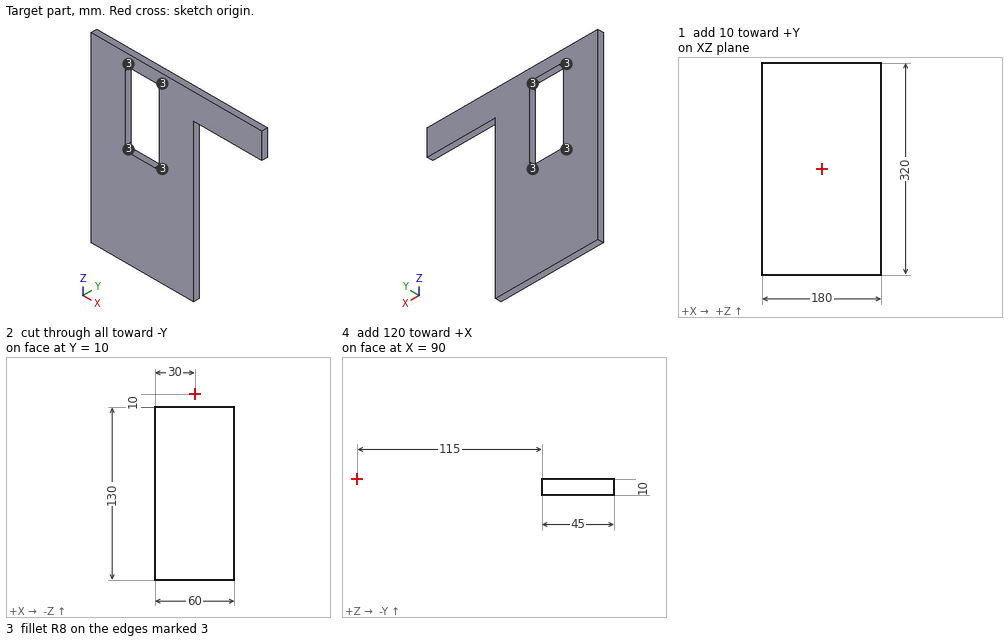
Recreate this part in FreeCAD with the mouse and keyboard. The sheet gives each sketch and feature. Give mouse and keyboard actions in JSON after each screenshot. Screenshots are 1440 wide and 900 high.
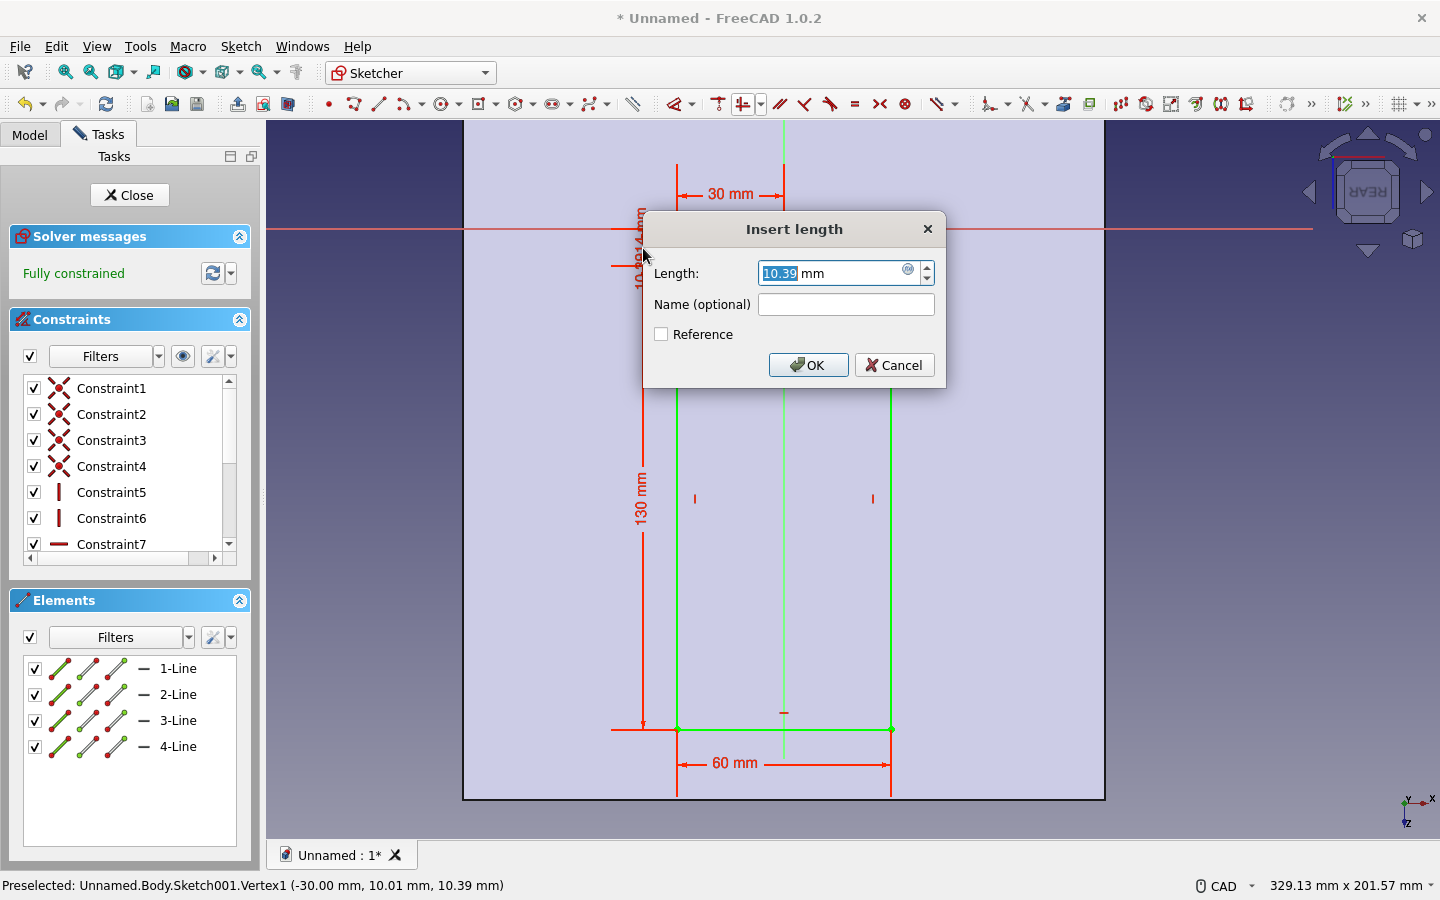
{"action": "type", "text": "10"}
{"action": "key", "text": "Return"}
{"action": "key", "text": "Escape"}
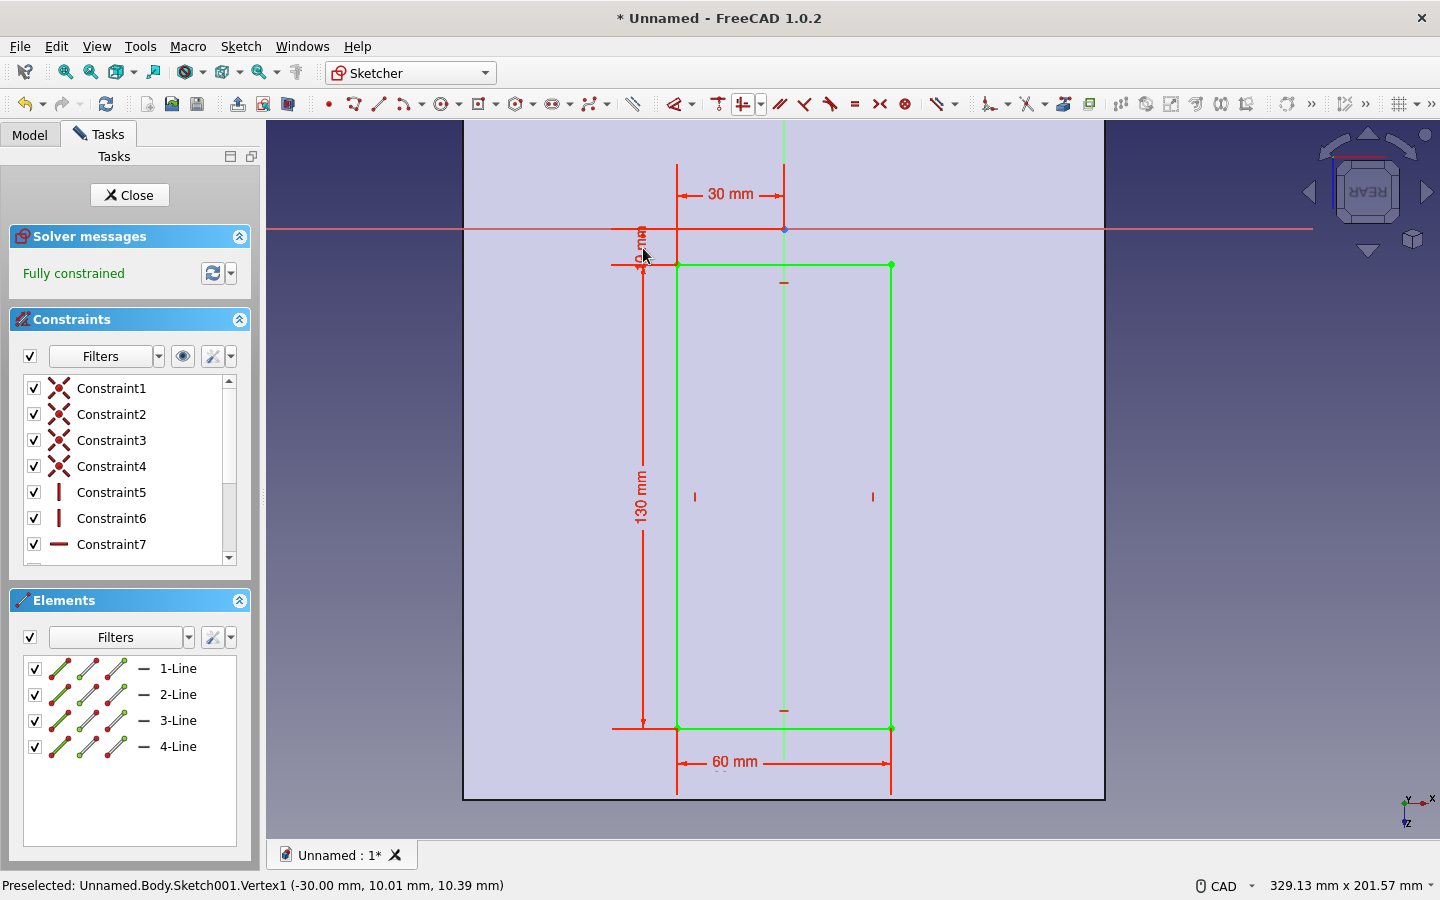
{"action": "left_click", "coordinate": [130, 195]}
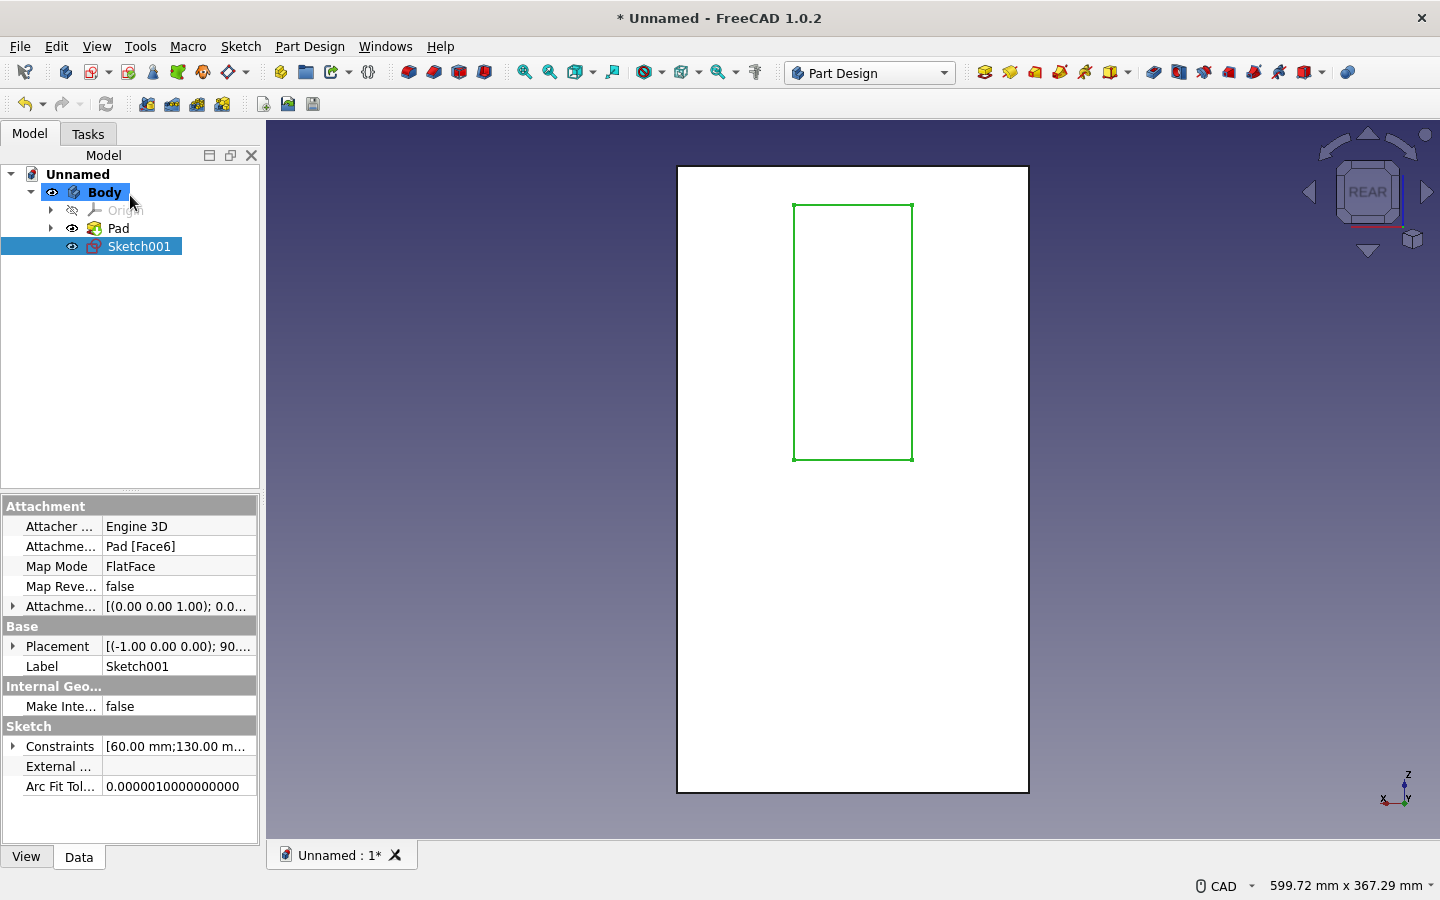
{"action": "left_click", "coordinate": [1154, 72]}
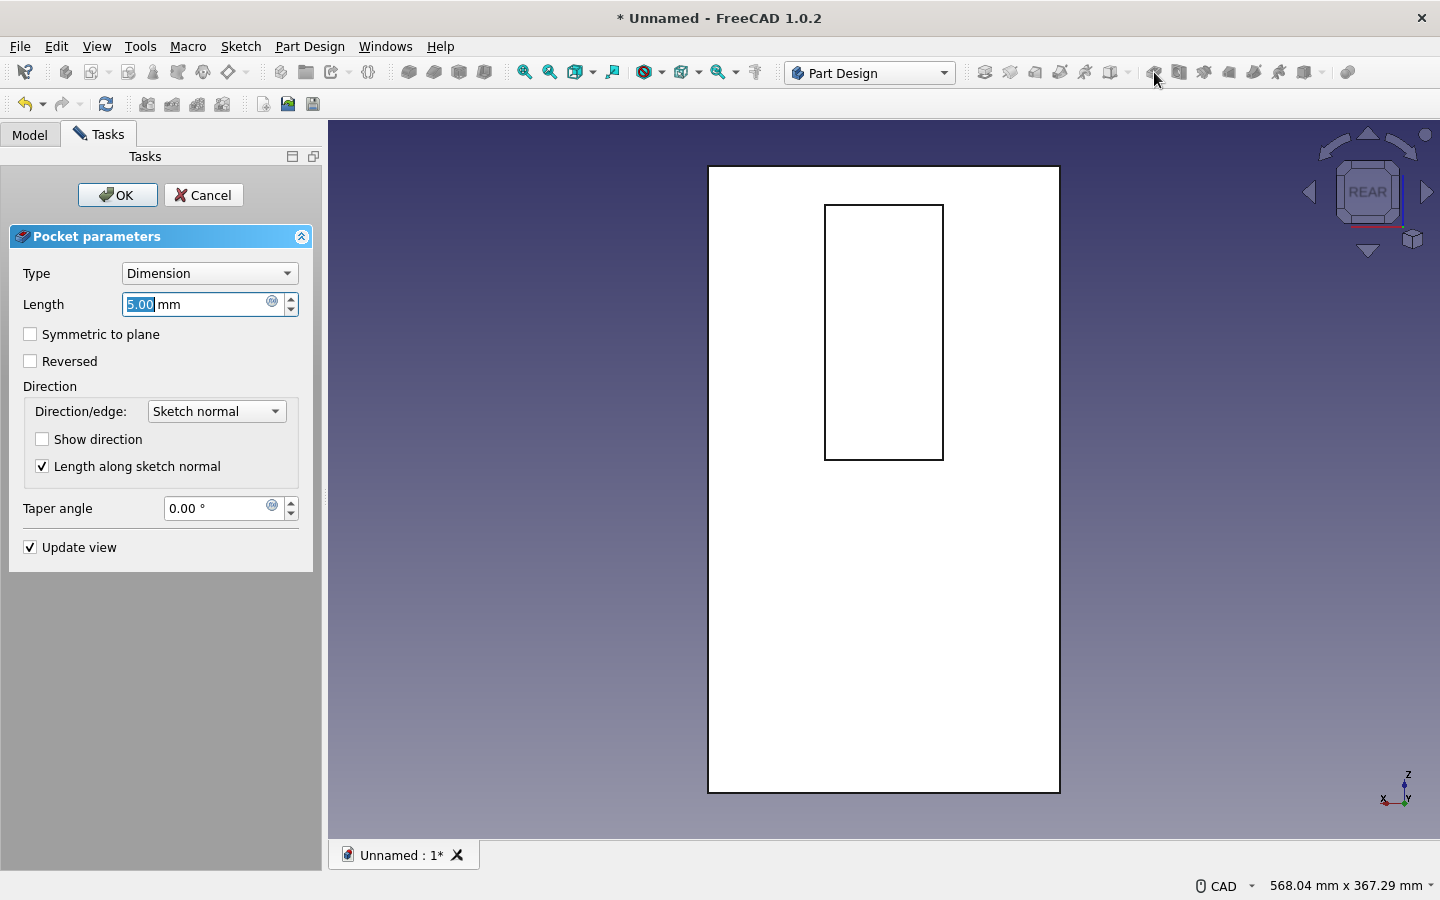
{"action": "left_click", "coordinate": [210, 274]}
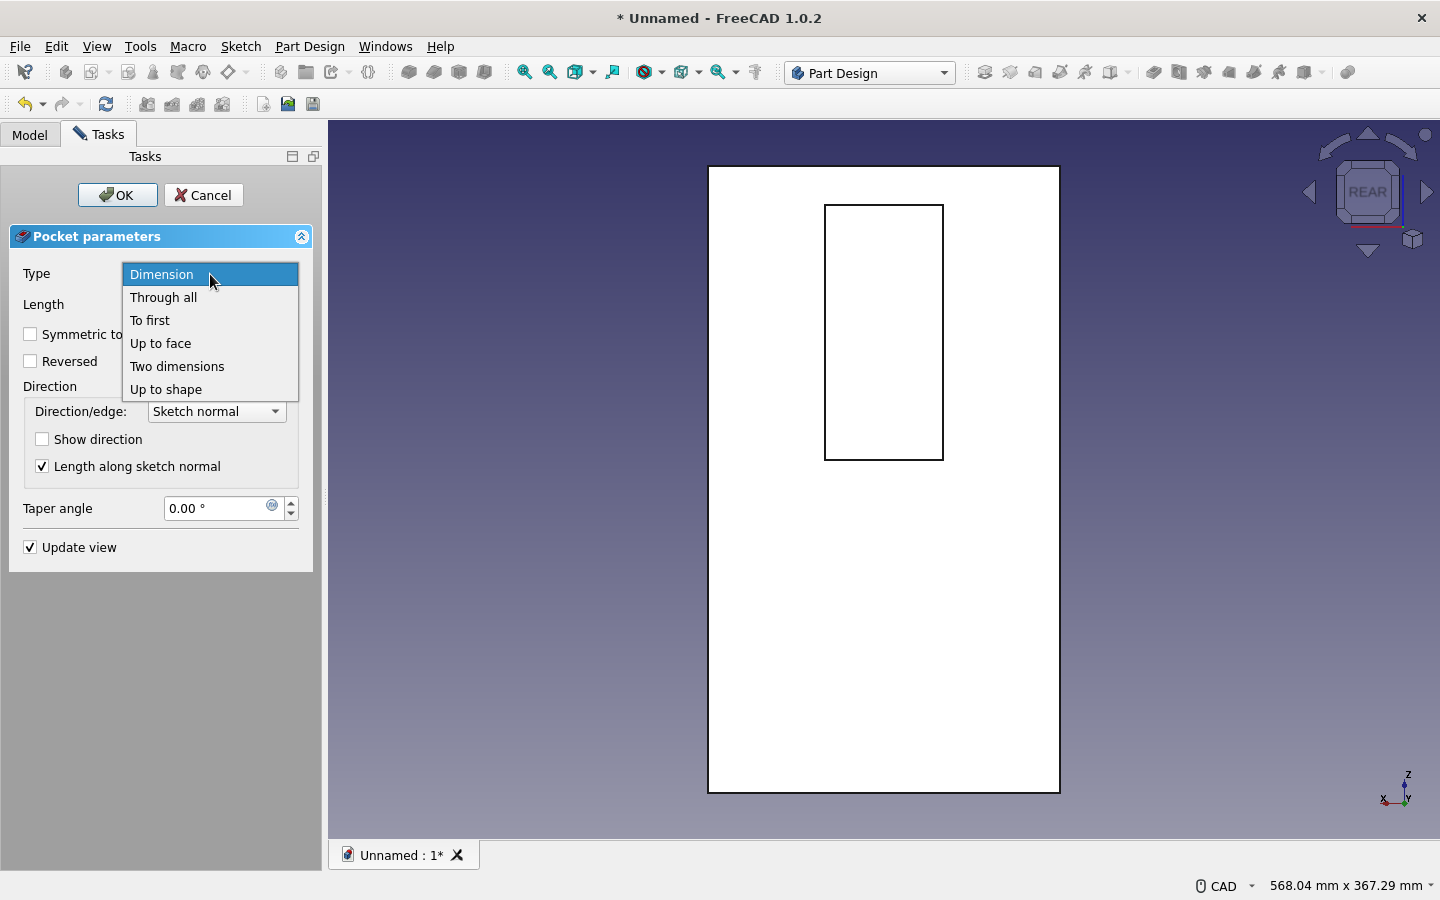
{"action": "left_click", "coordinate": [208, 298]}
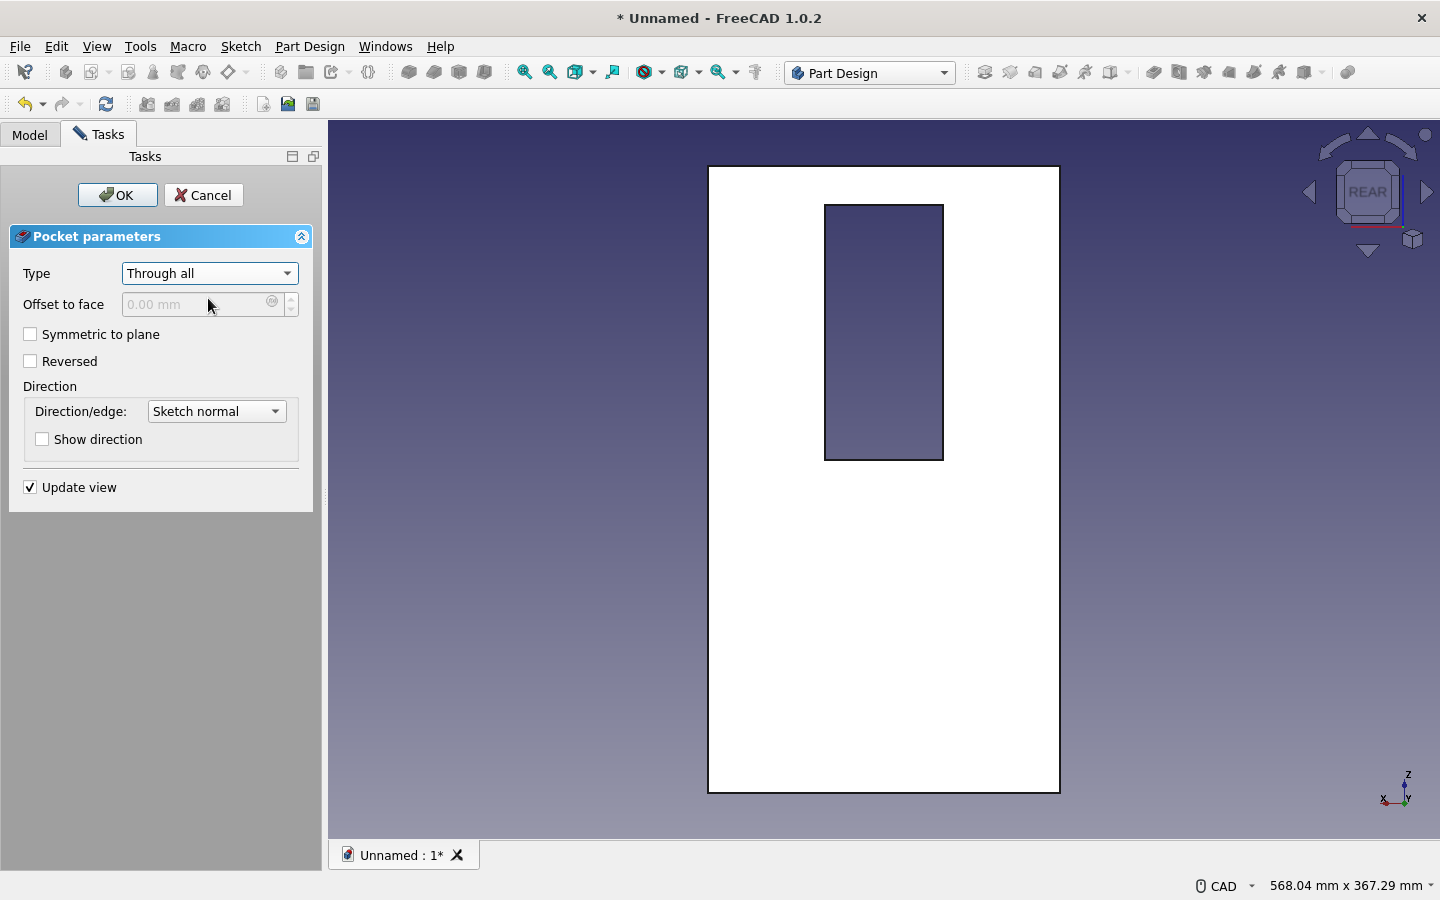
{"action": "left_click", "coordinate": [118, 195]}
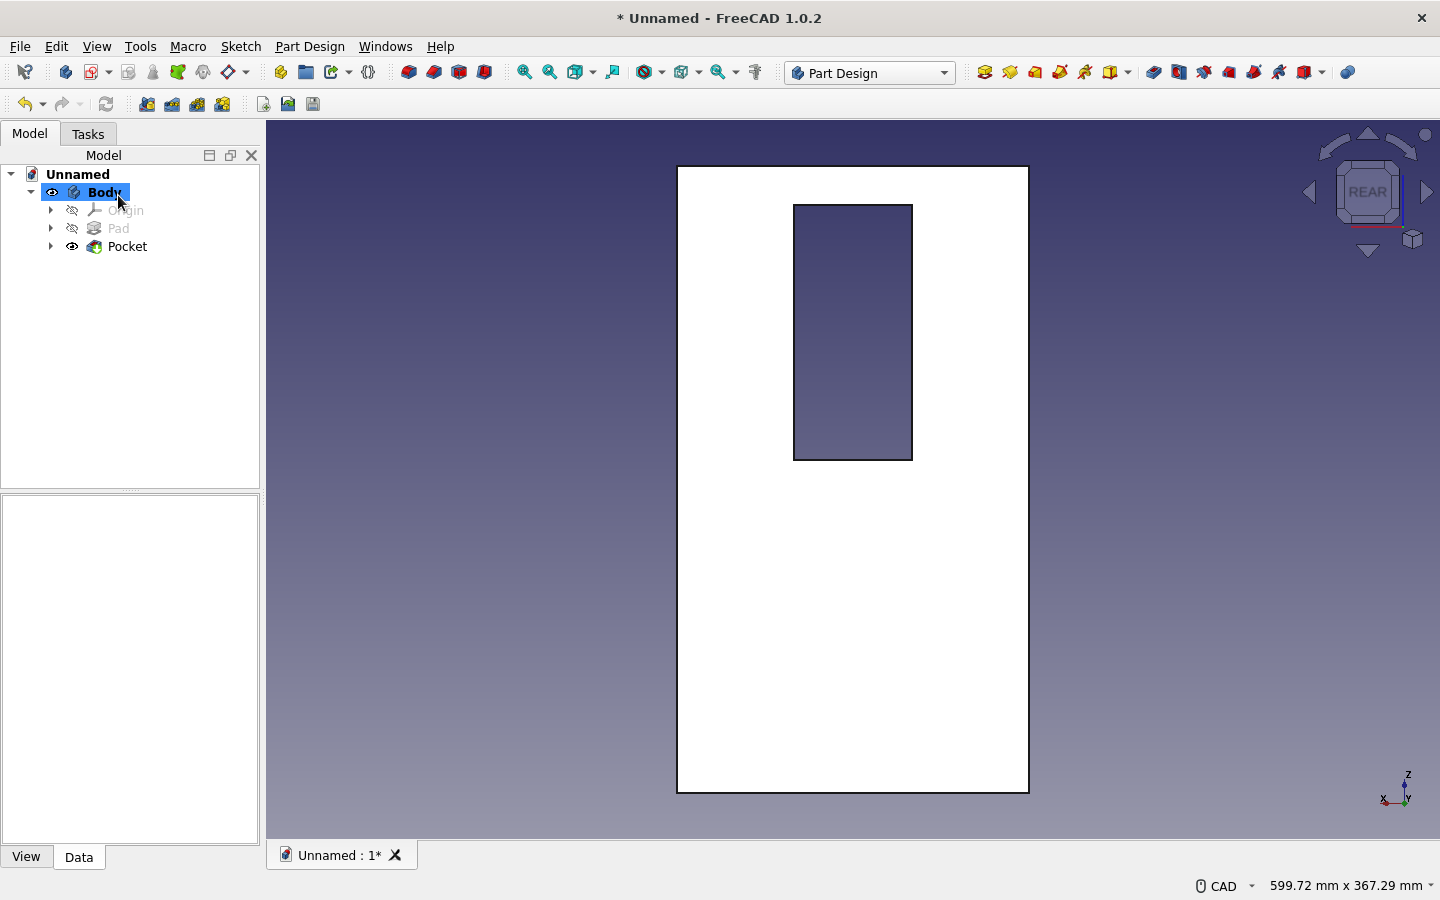
{"action": "scroll", "coordinate": [794, 459], "scroll_direction": "up", "scroll_amount": 4}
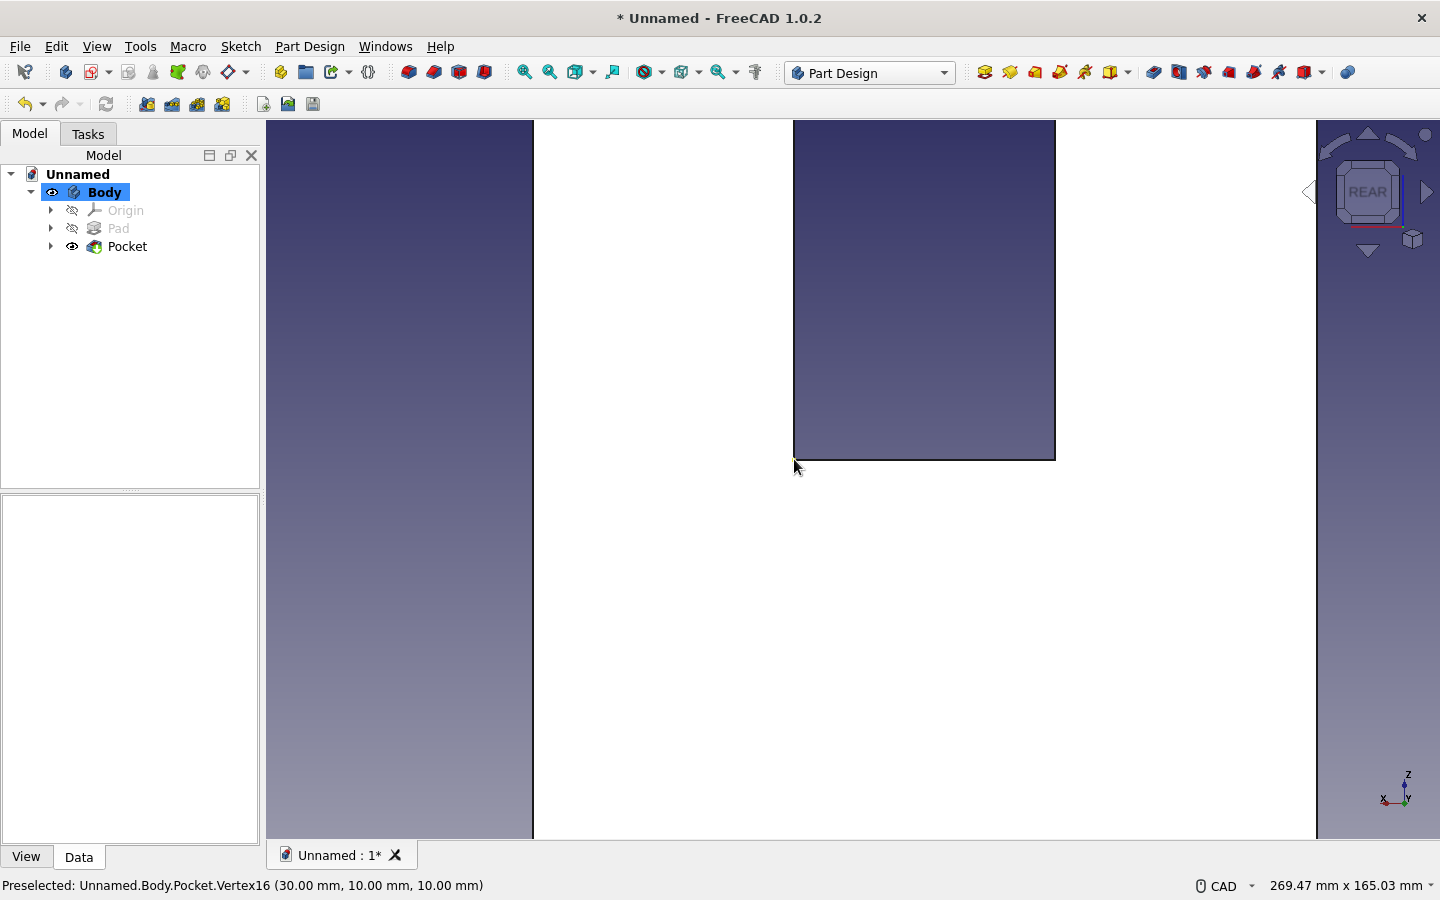
{"action": "key", "text": "v f"}